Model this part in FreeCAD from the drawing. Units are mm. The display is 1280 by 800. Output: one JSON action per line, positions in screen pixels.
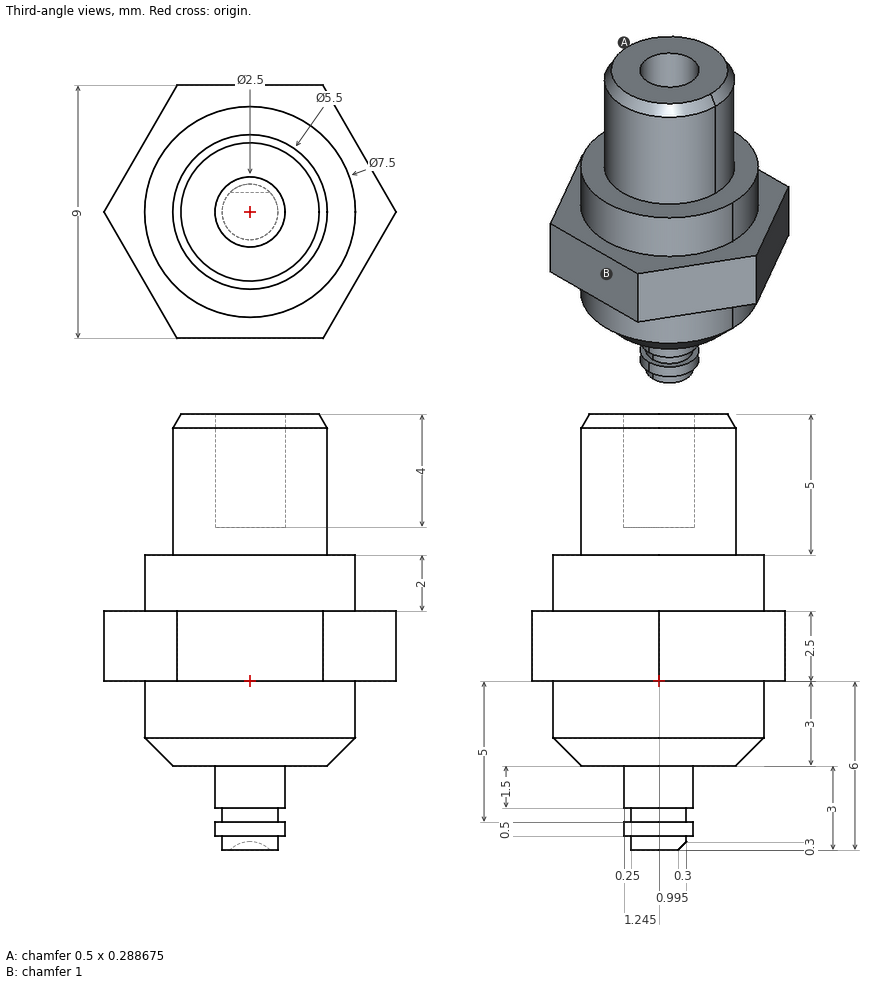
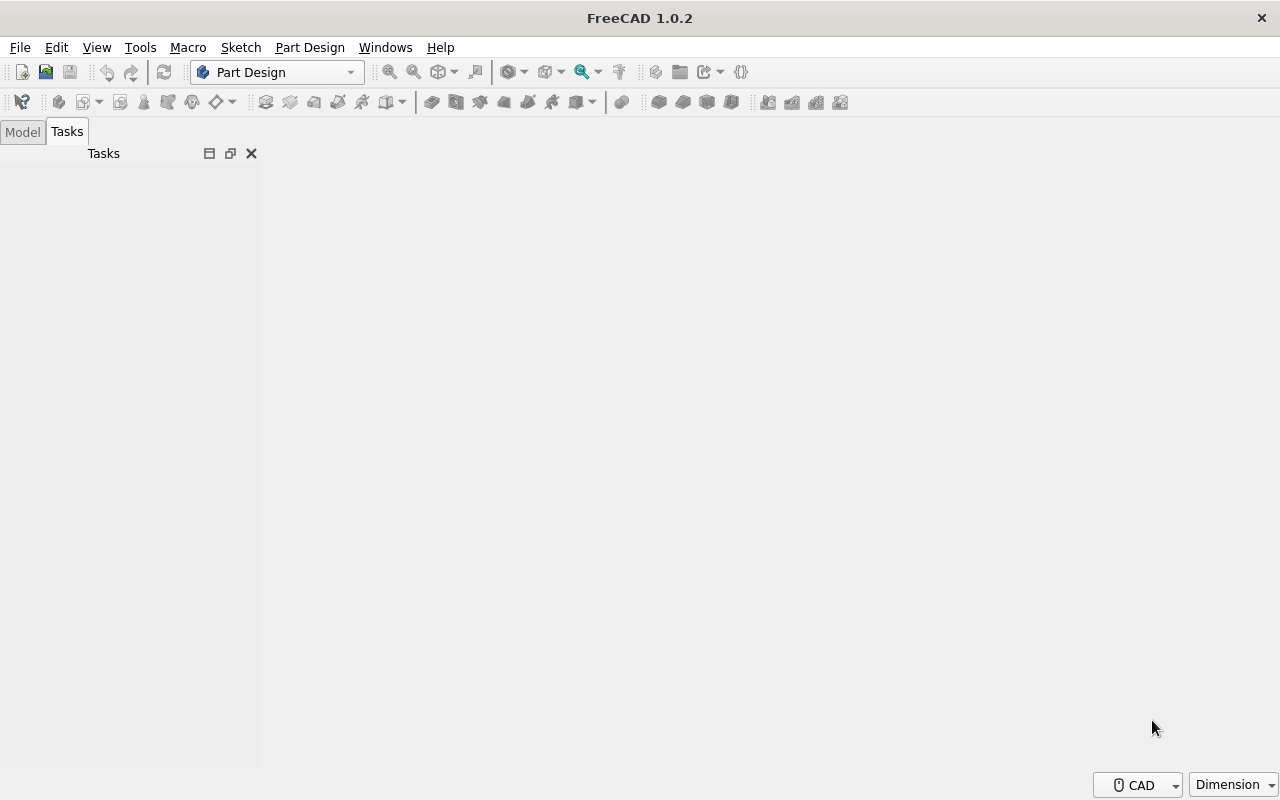
{"action": "key", "text": "ctrl+n"}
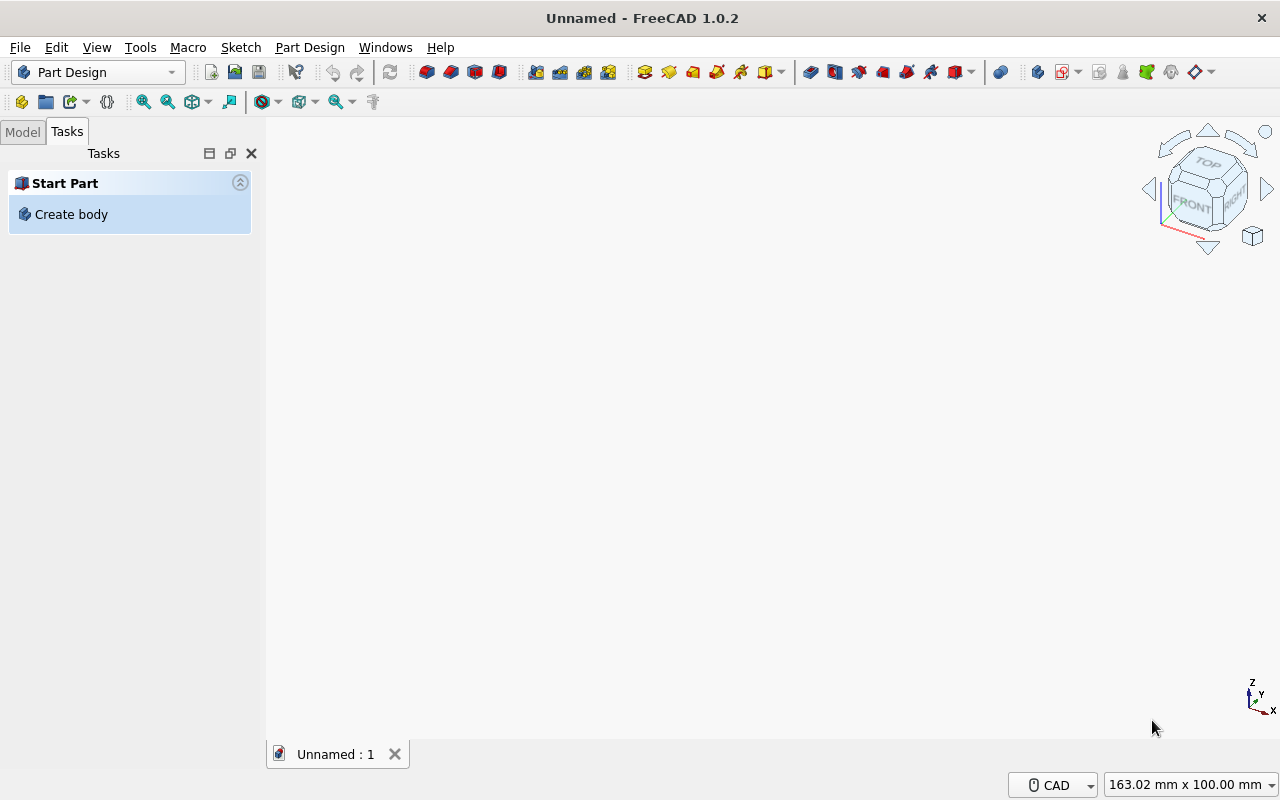
{"action": "left_click", "coordinate": [1062, 72]}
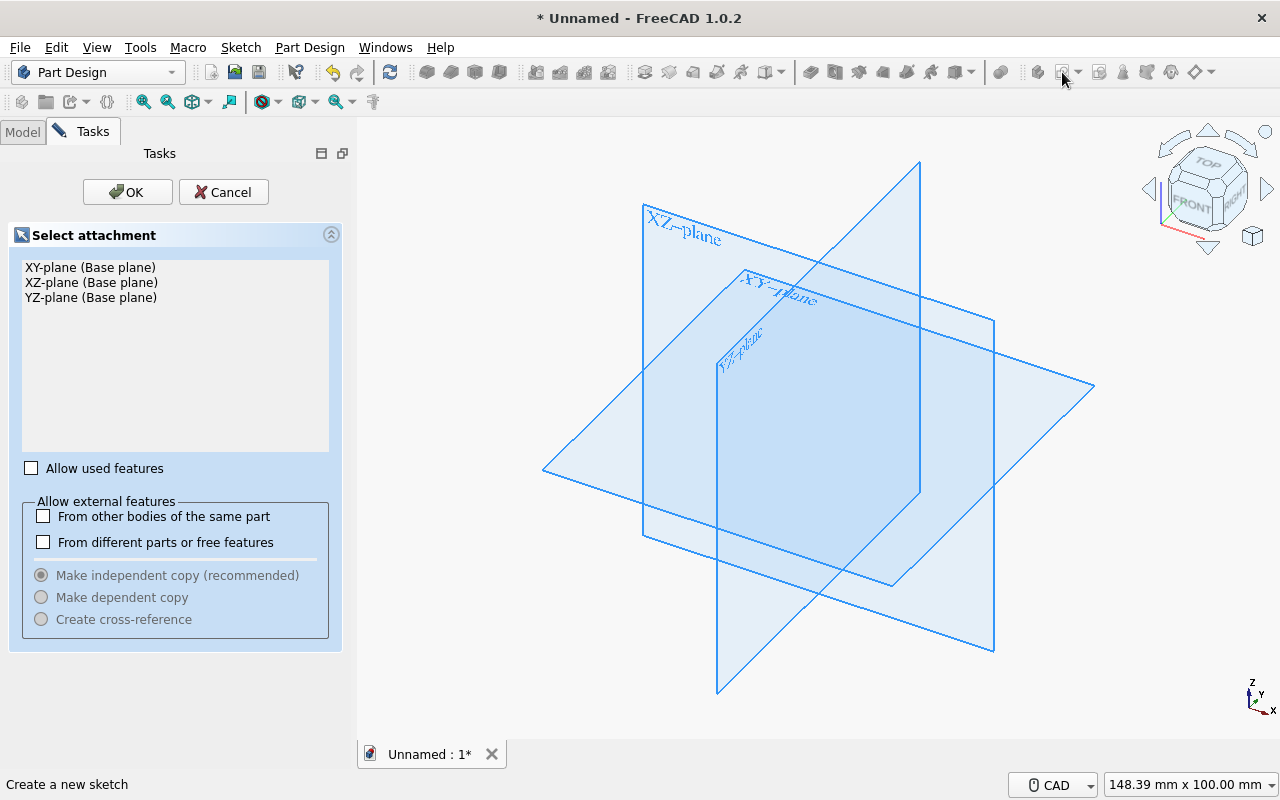
{"action": "left_click", "coordinate": [82, 268]}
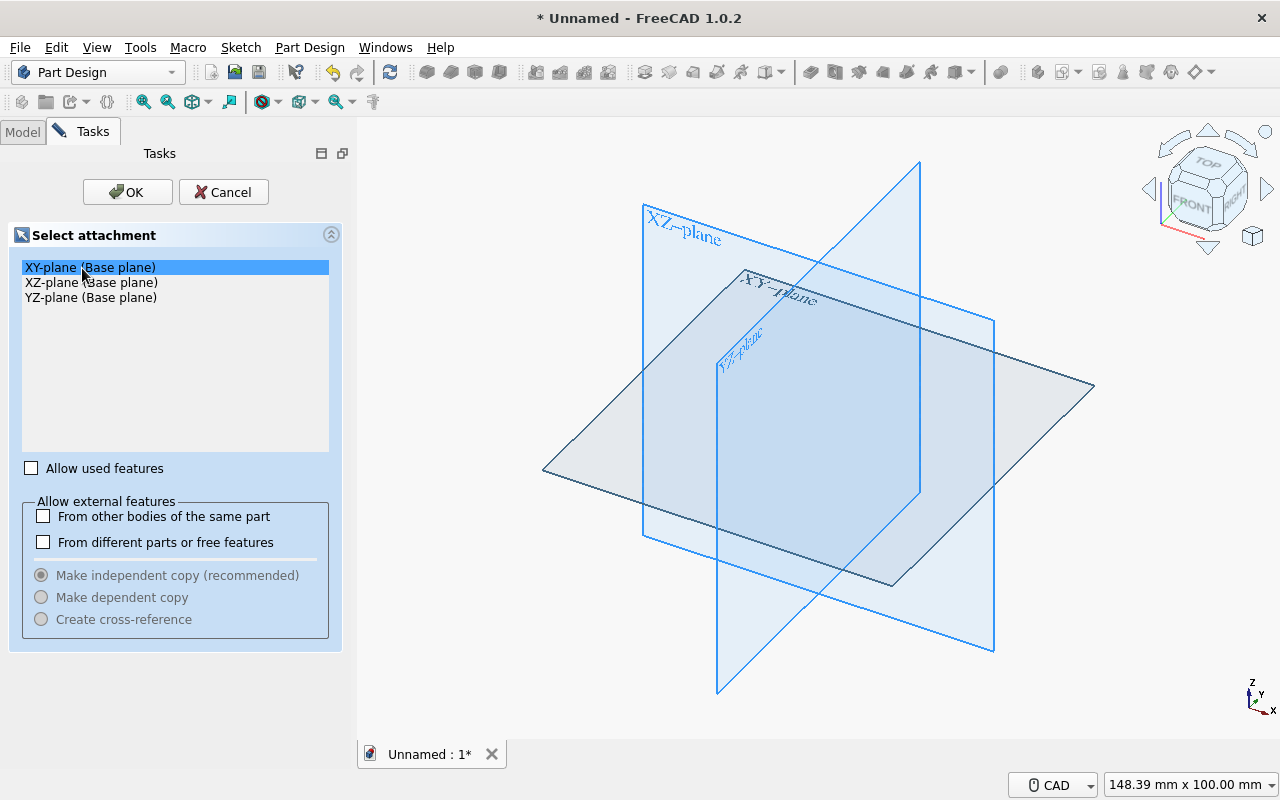
{"action": "left_click", "coordinate": [128, 192]}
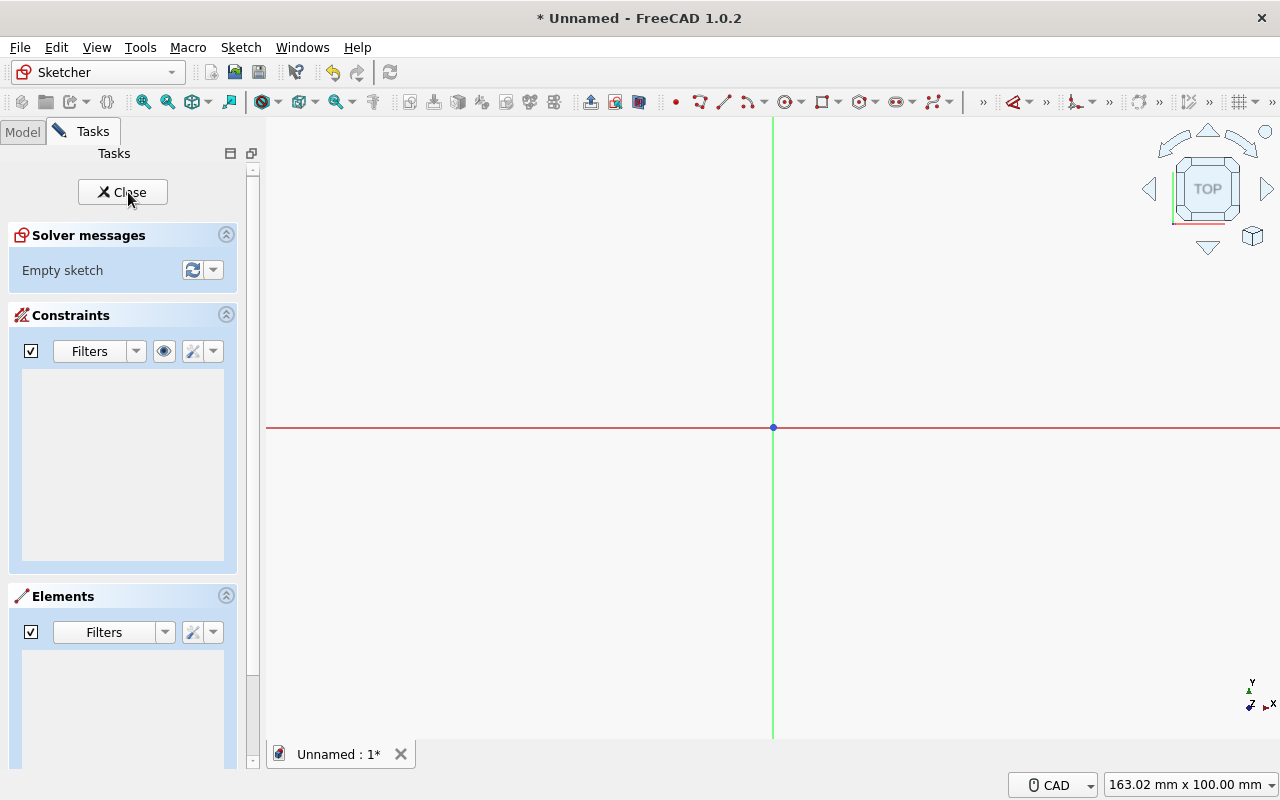
{"action": "scroll", "coordinate": [784, 428], "scroll_direction": "up", "scroll_amount": 10}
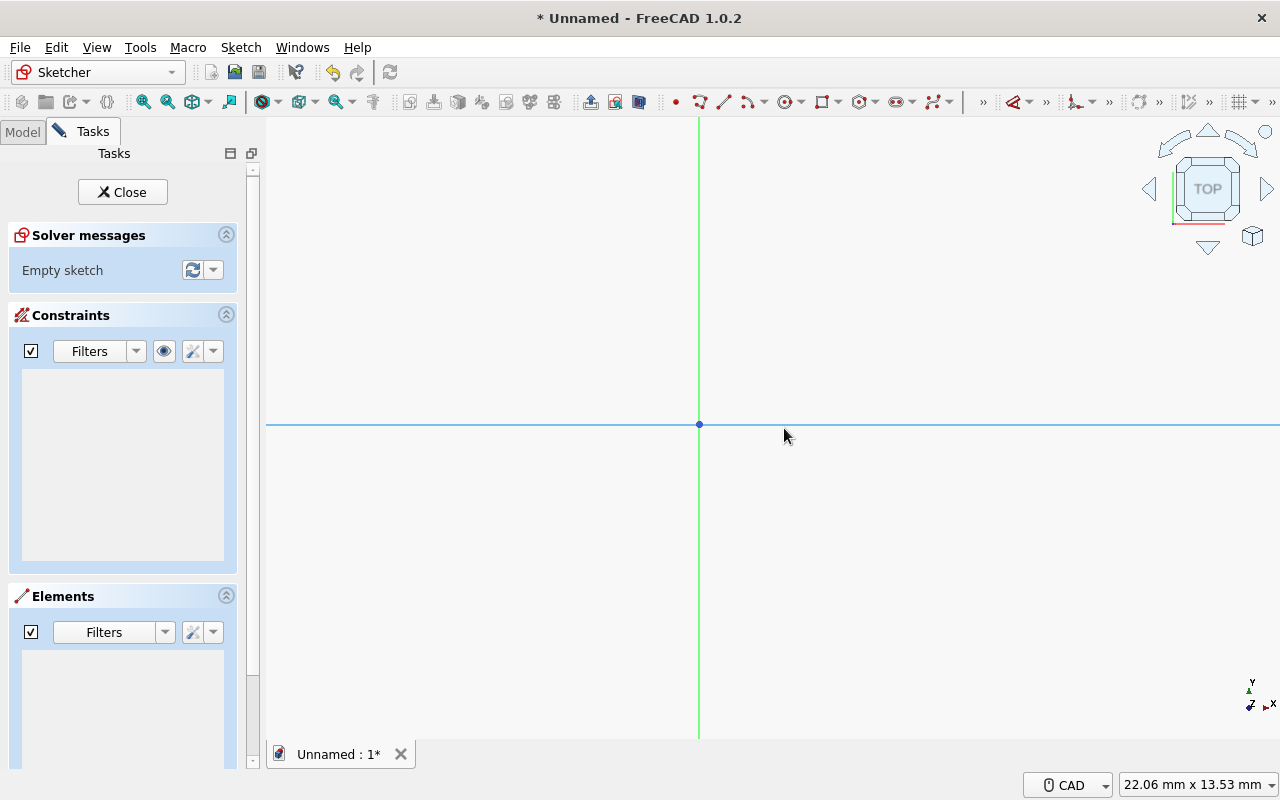
{"action": "left_click", "coordinate": [860, 102]}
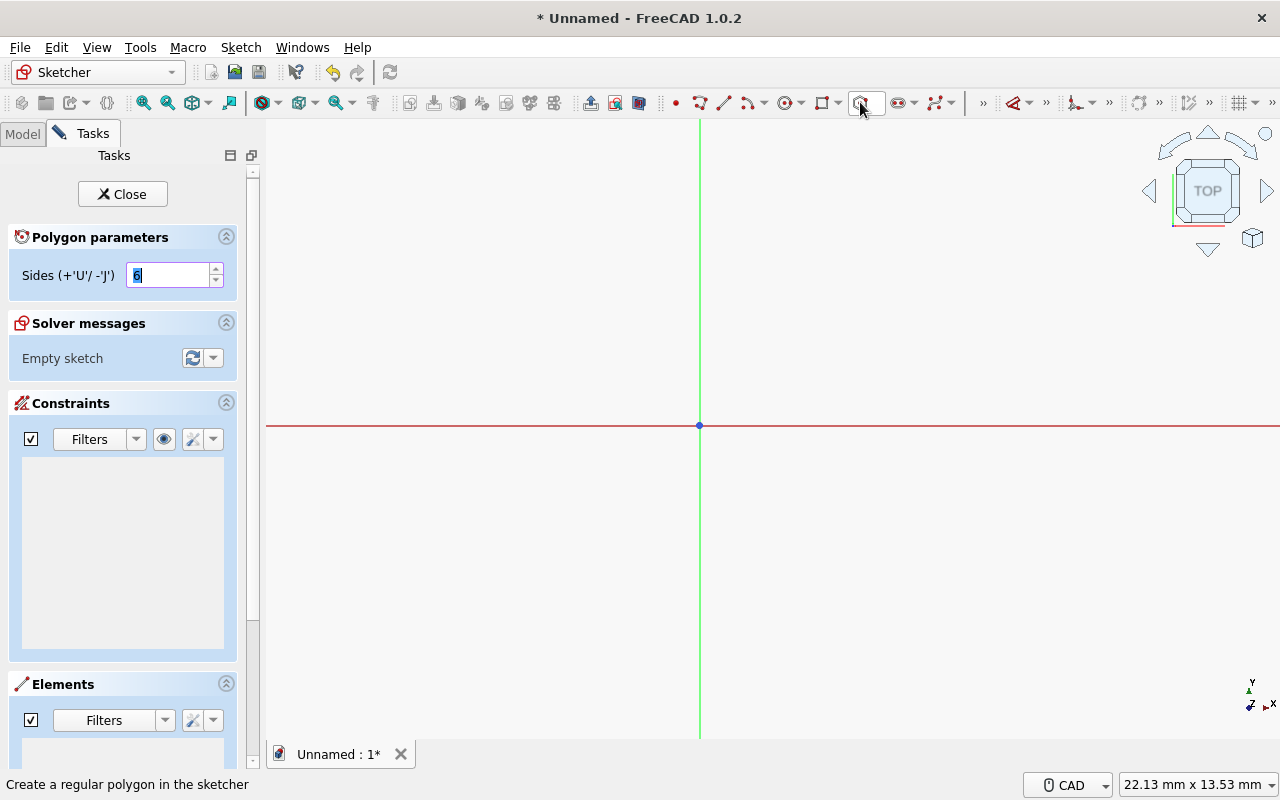
{"action": "left_click", "coordinate": [700, 426]}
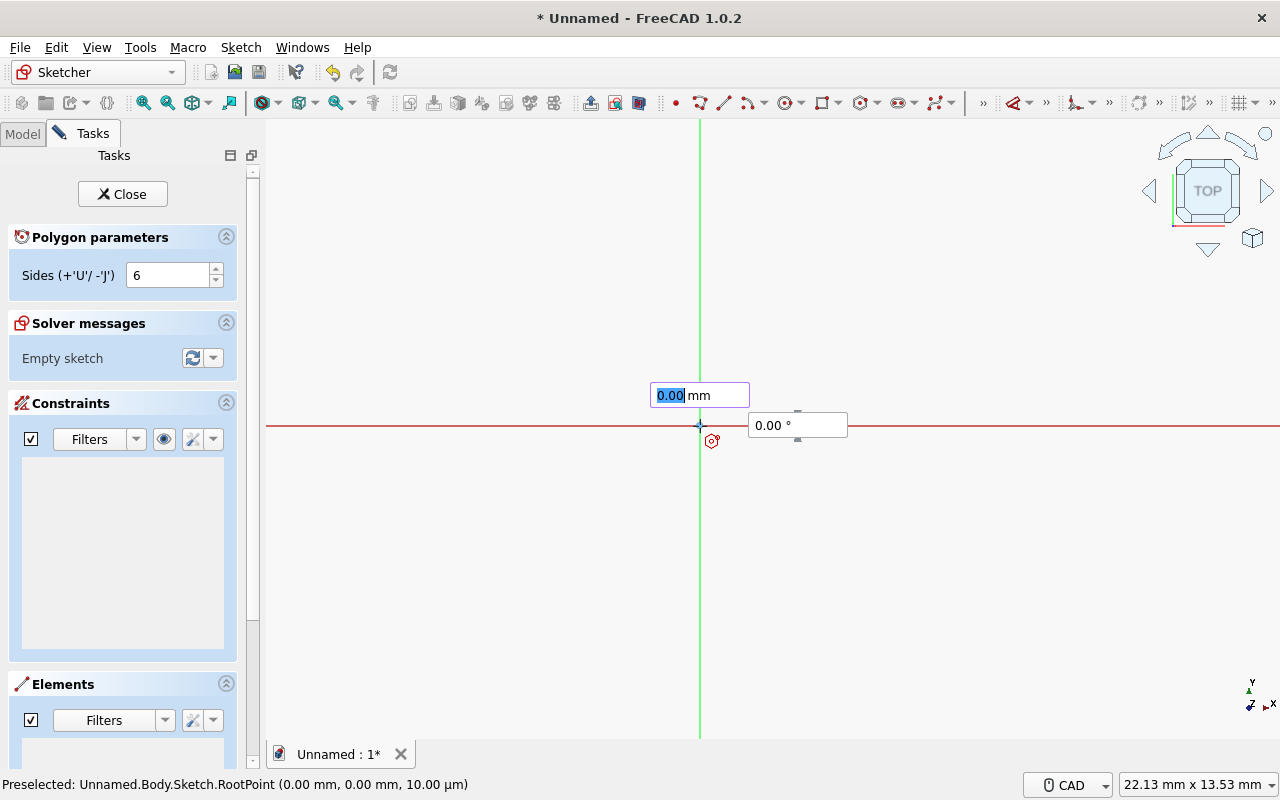
{"action": "left_click", "coordinate": [462, 426]}
{"action": "key", "text": "Escape"}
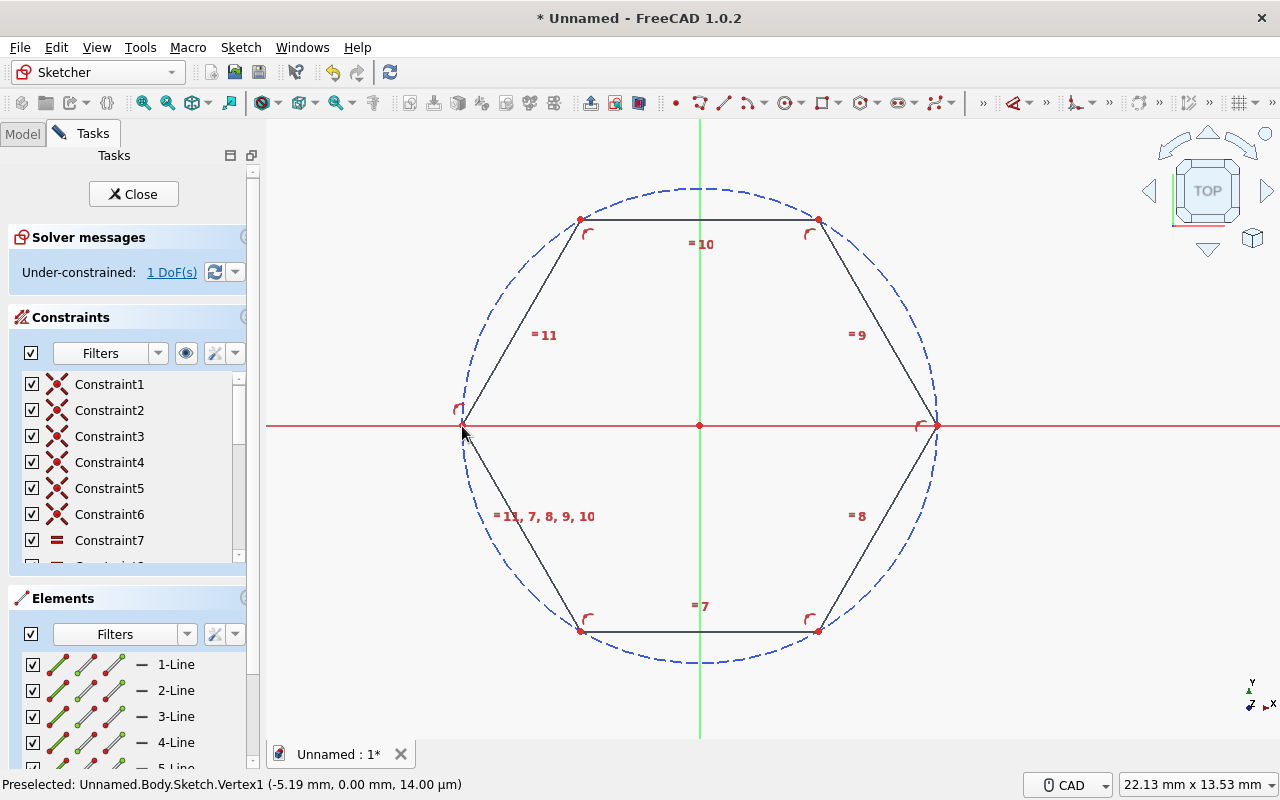
{"action": "left_click", "coordinate": [581, 632]}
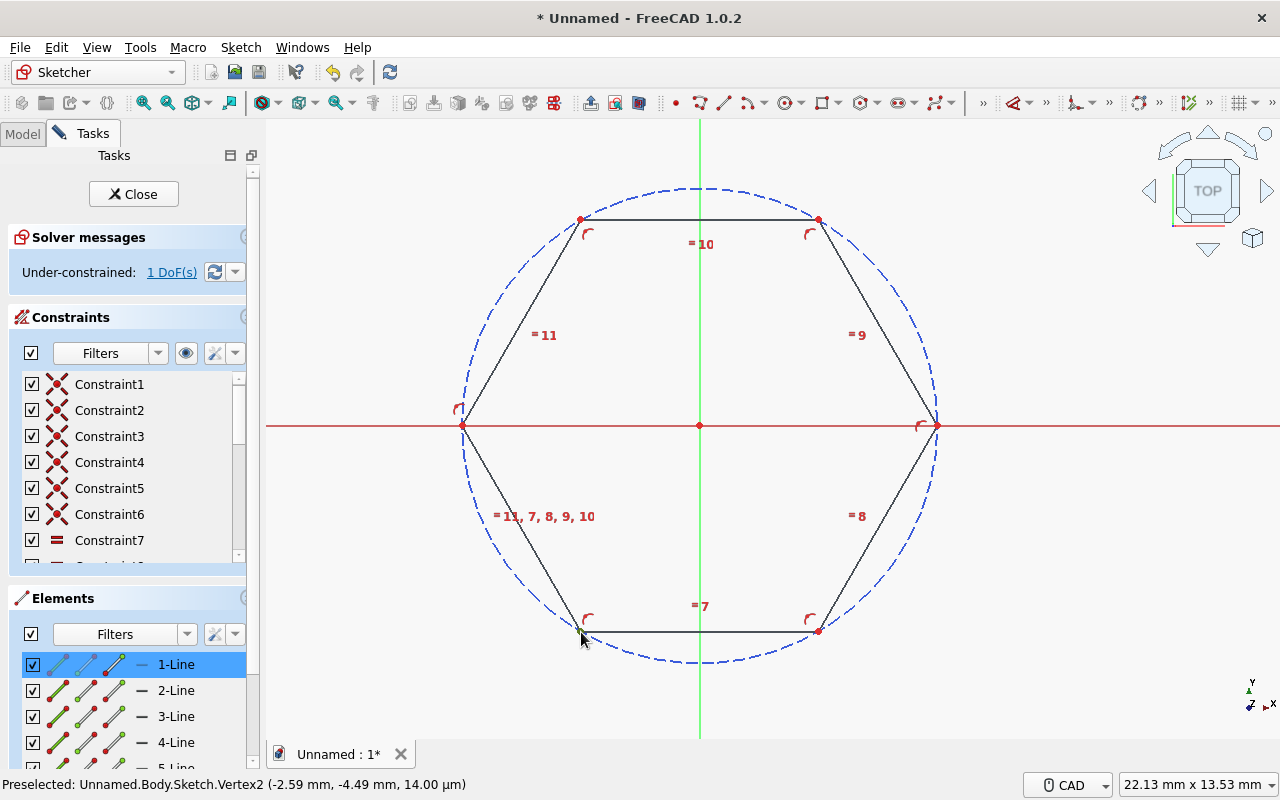
{"action": "left_click", "coordinate": [819, 220]}